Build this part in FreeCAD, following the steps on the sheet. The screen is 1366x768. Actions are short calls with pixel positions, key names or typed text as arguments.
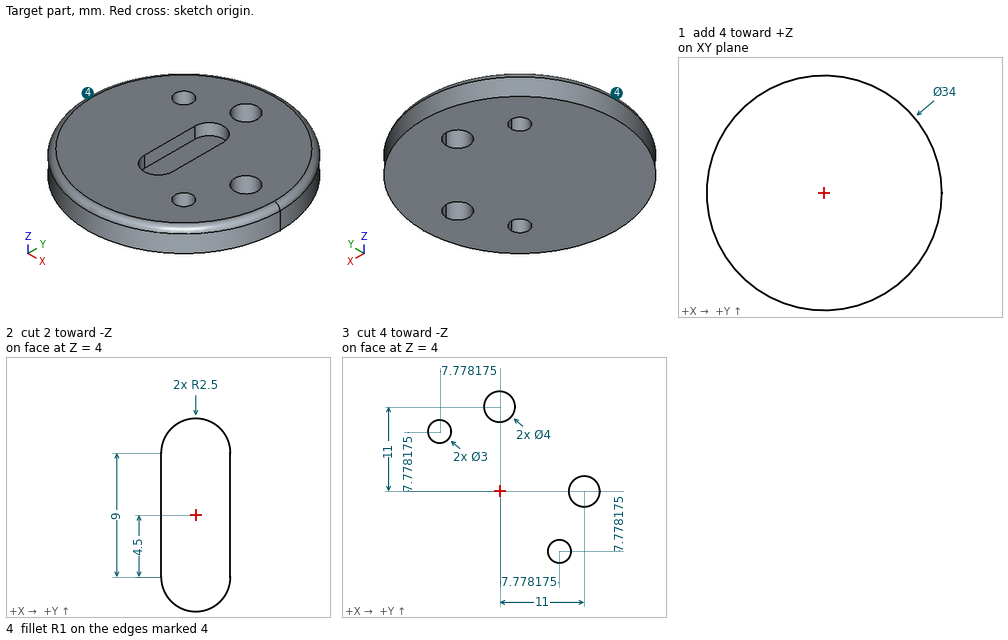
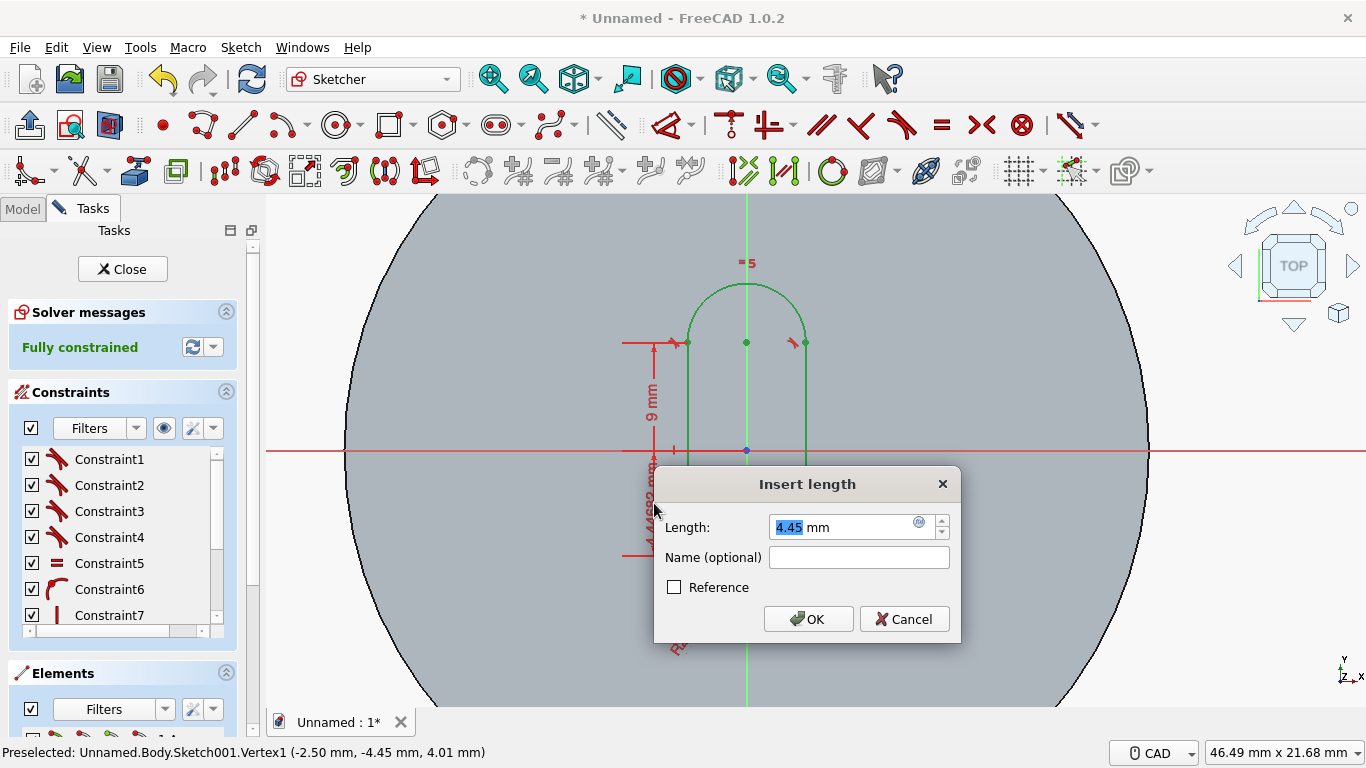
text(4.5)
key(Return)
key(Escape)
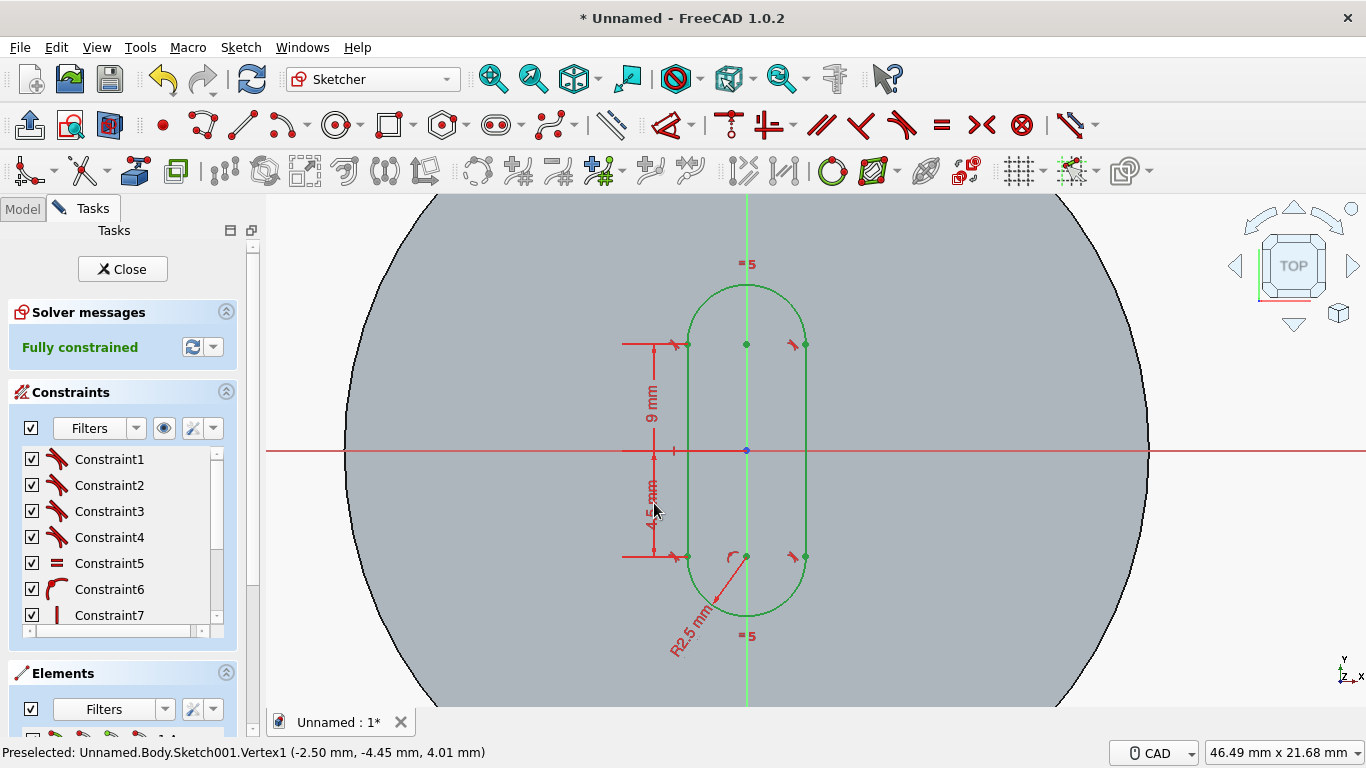
click(123, 269)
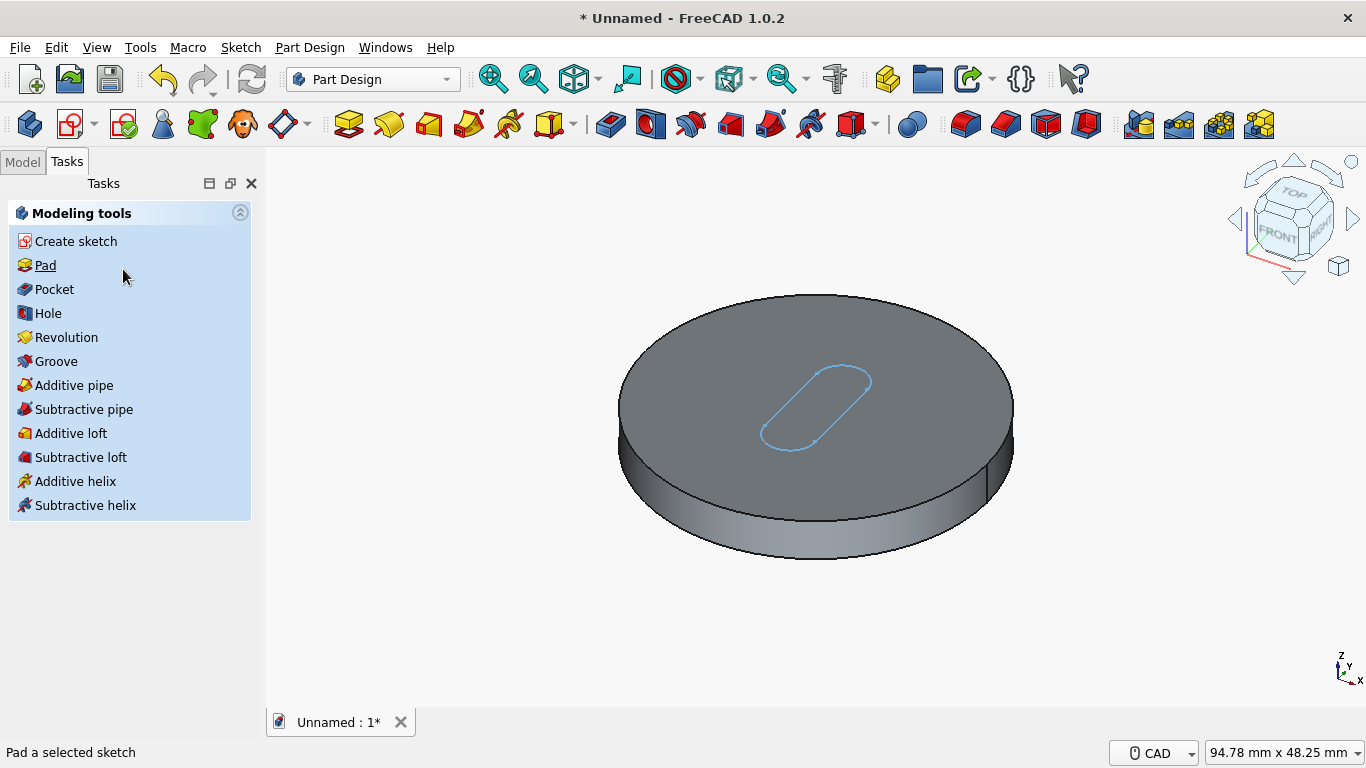
click(612, 124)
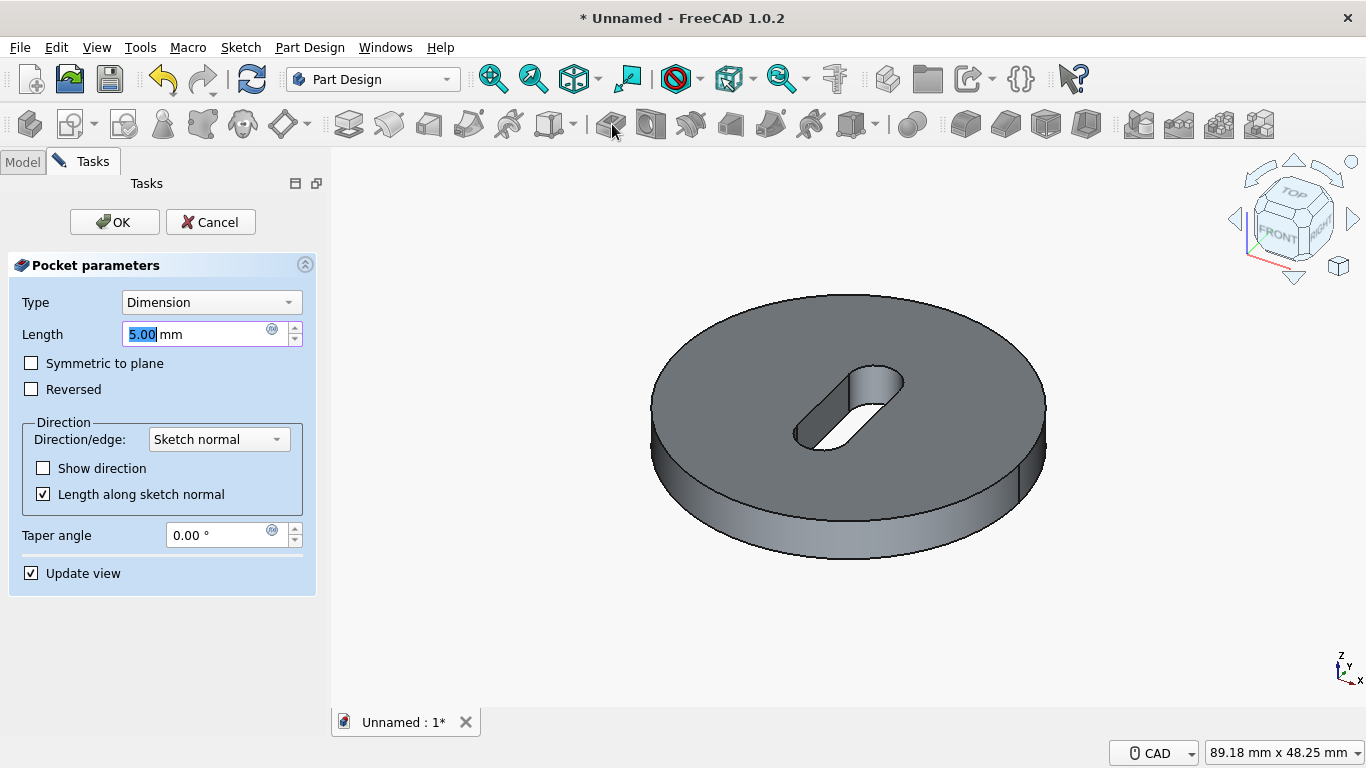
text(2)
key(Tab)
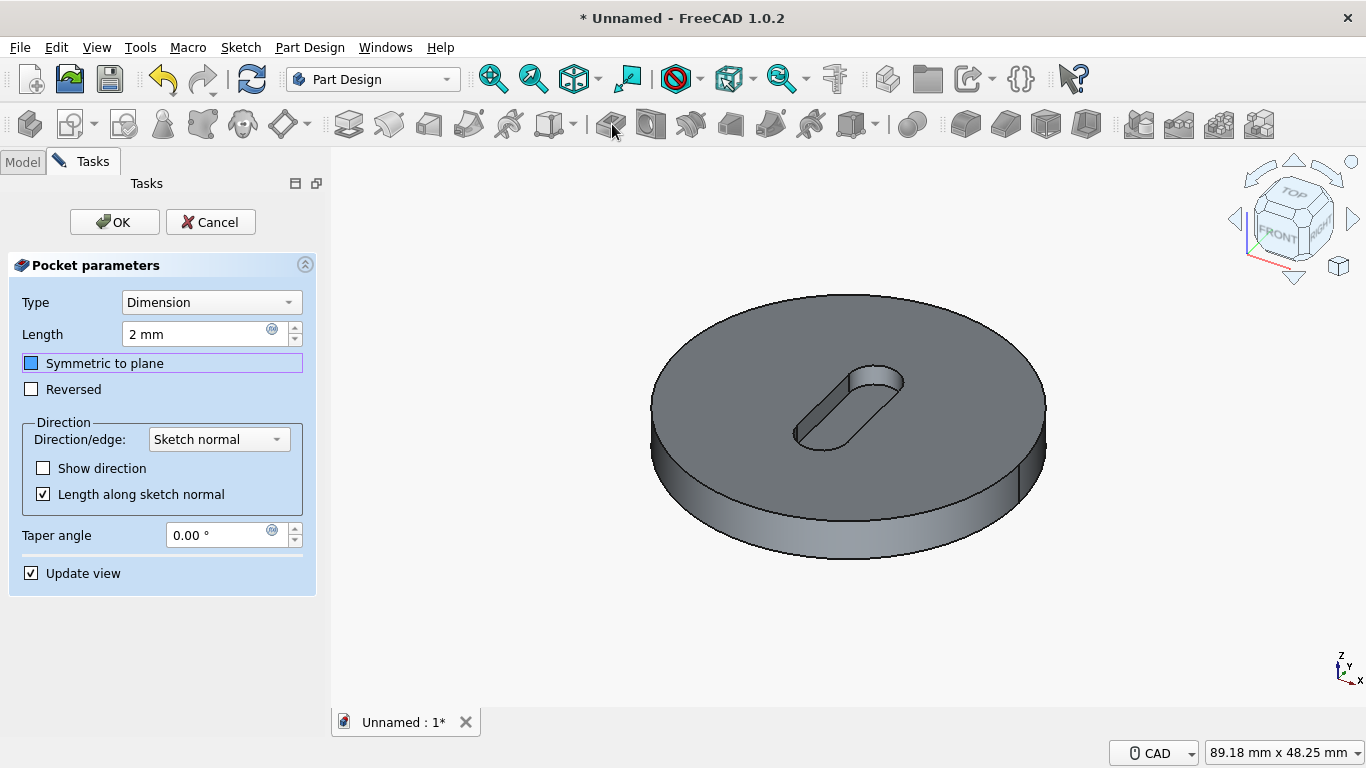
click(115, 222)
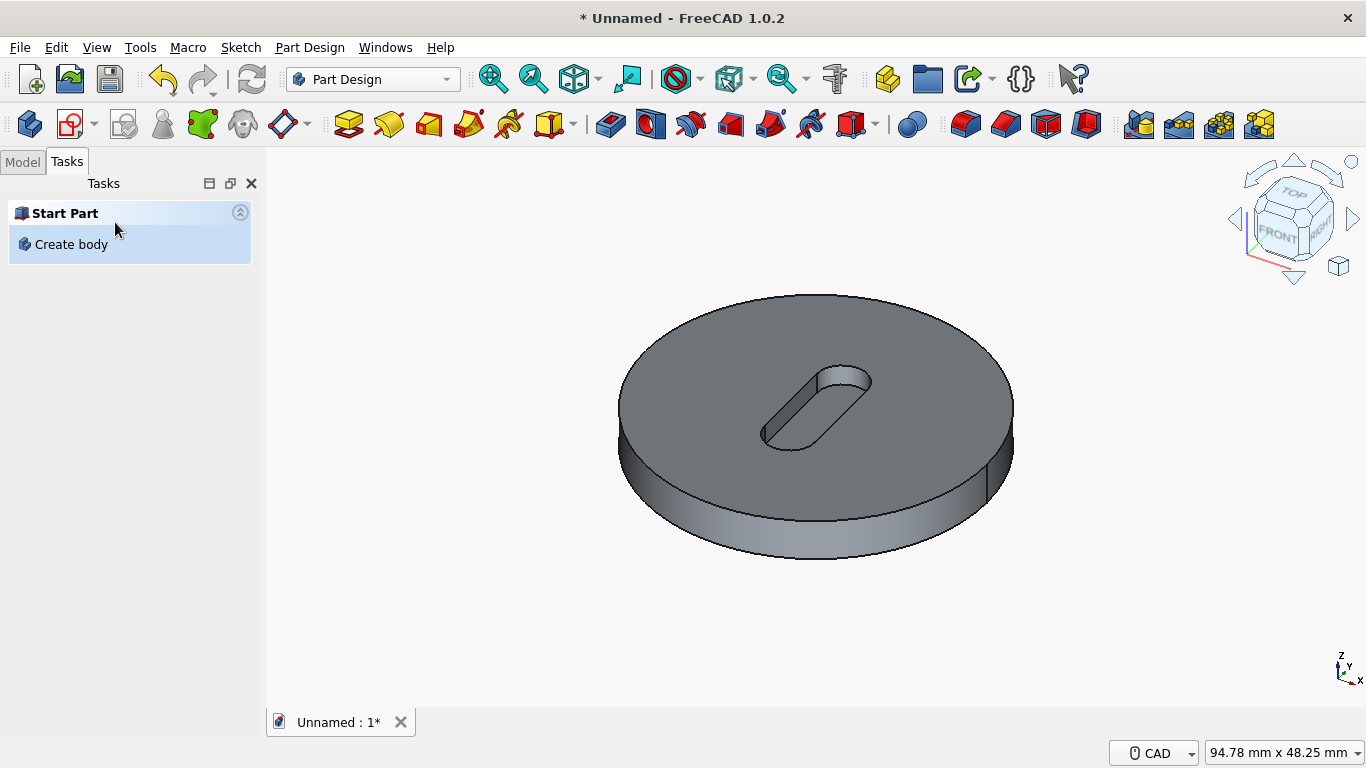
click(718, 375)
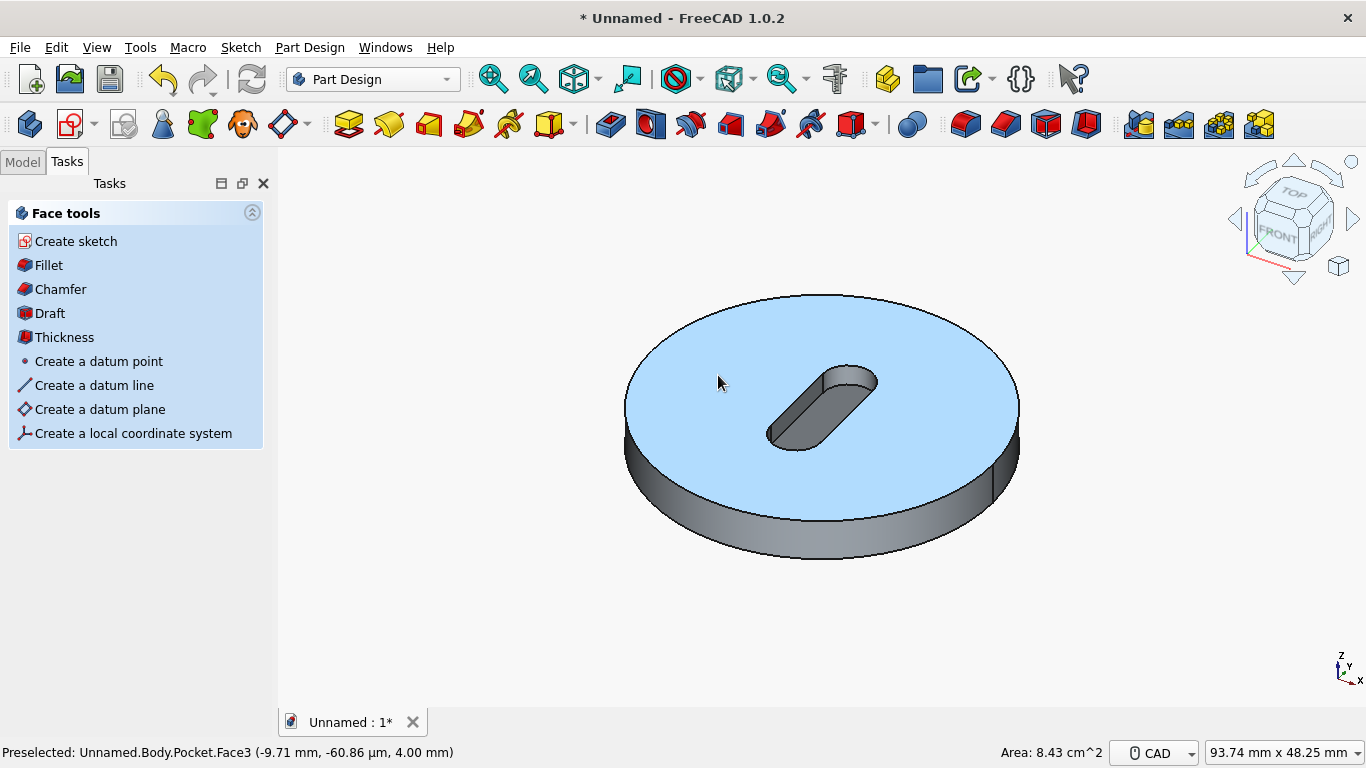
click(70, 124)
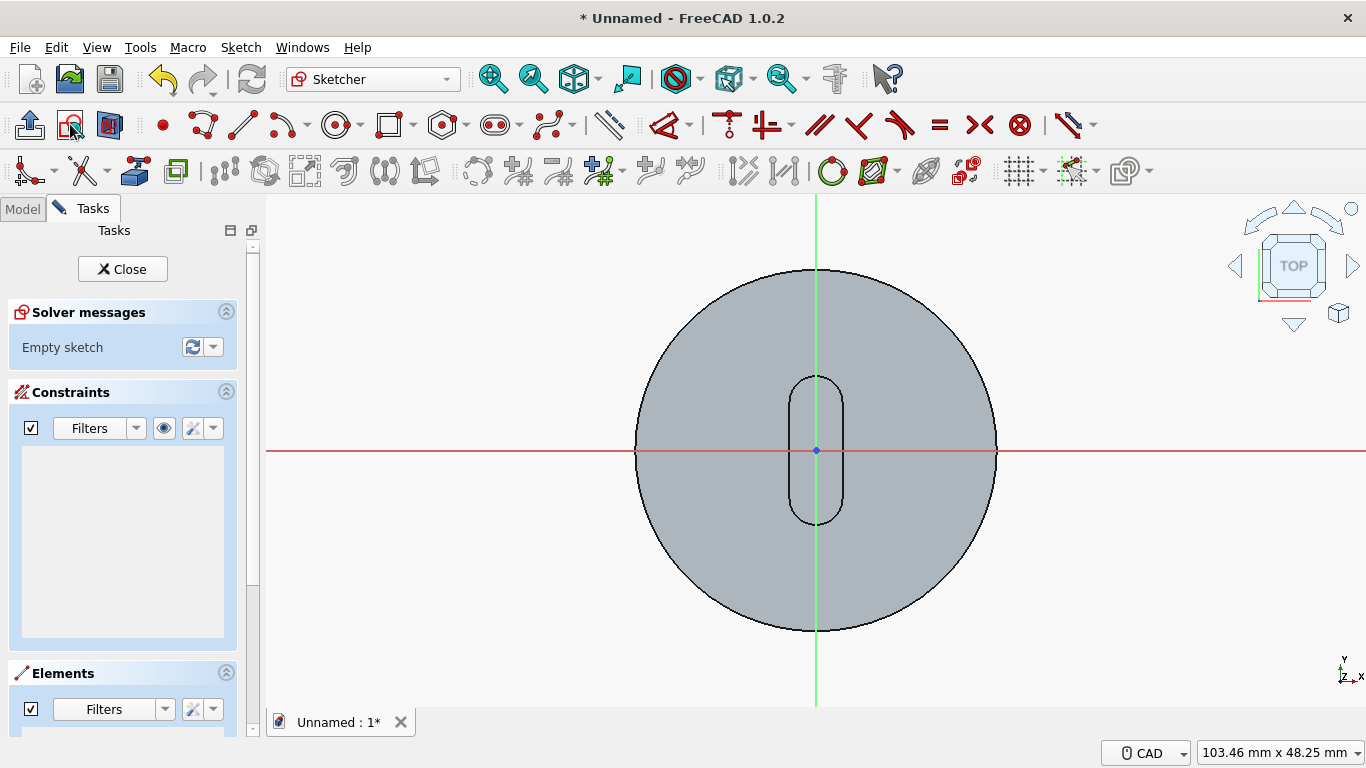
scroll(1015, 390, up, 2)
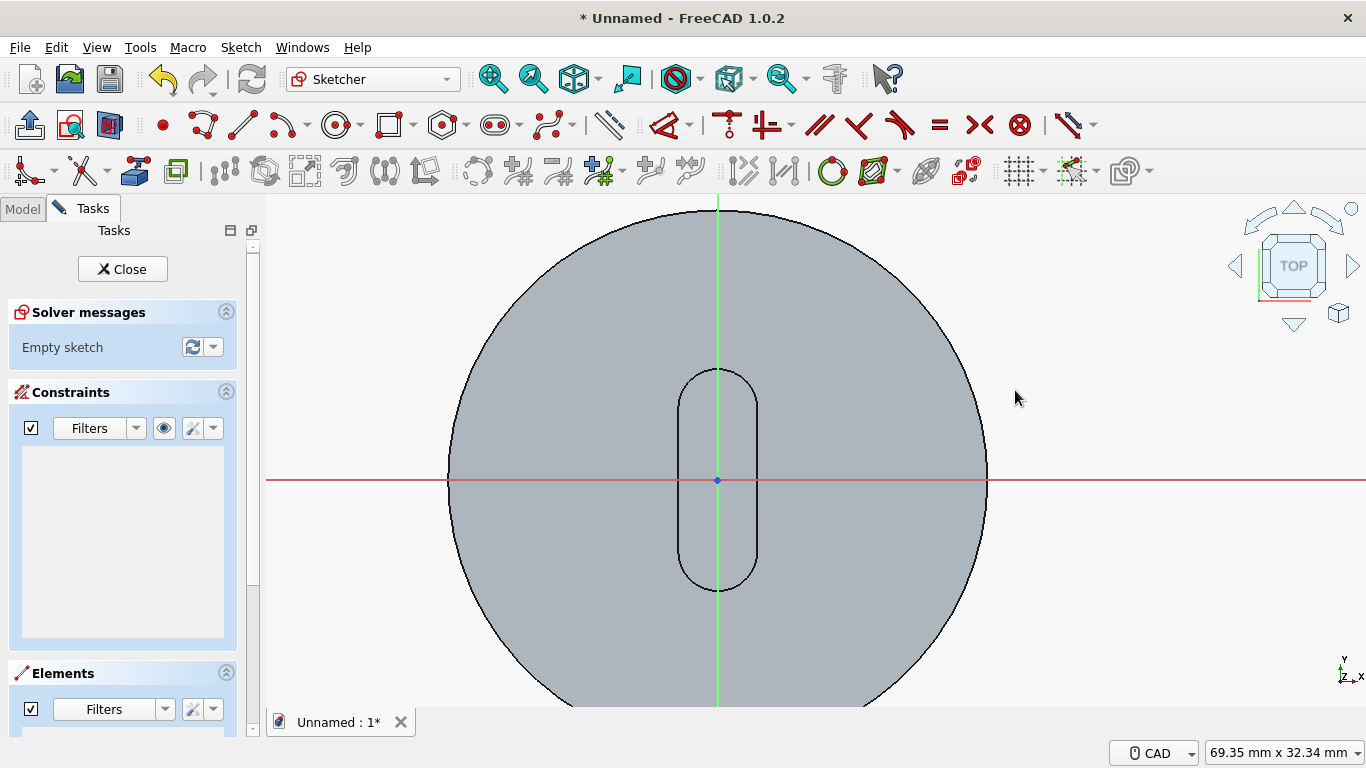
key(g)
key(c)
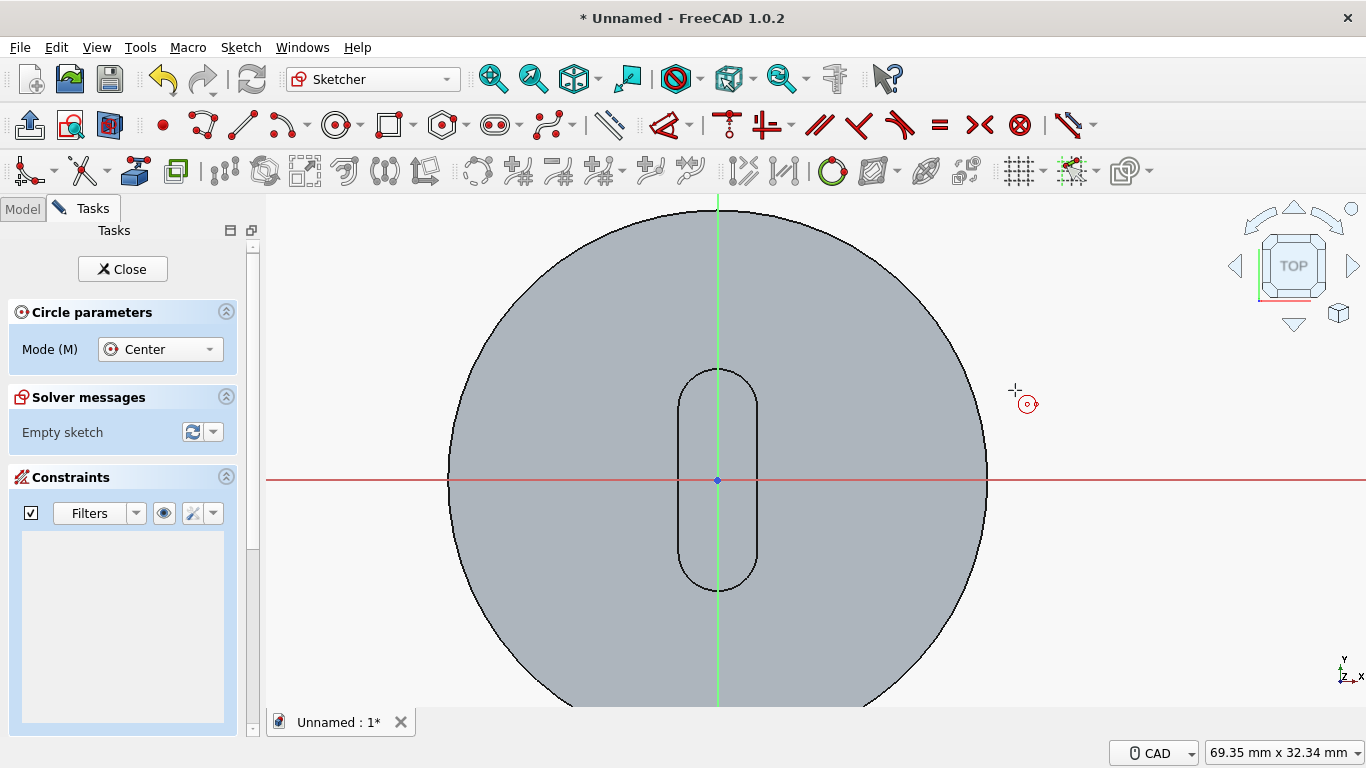
click(718, 306)
click(740, 283)